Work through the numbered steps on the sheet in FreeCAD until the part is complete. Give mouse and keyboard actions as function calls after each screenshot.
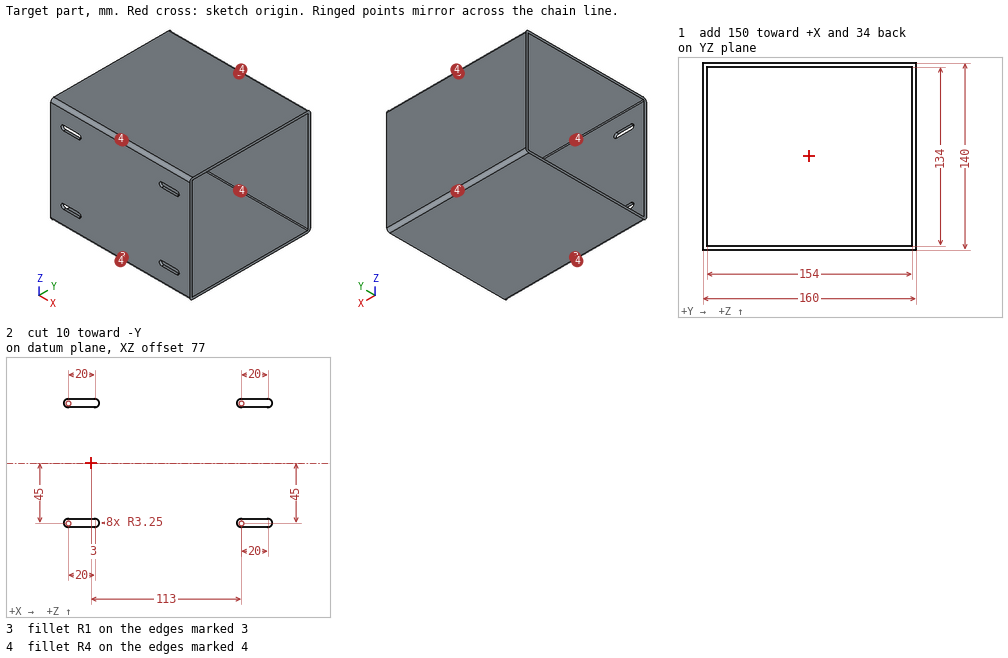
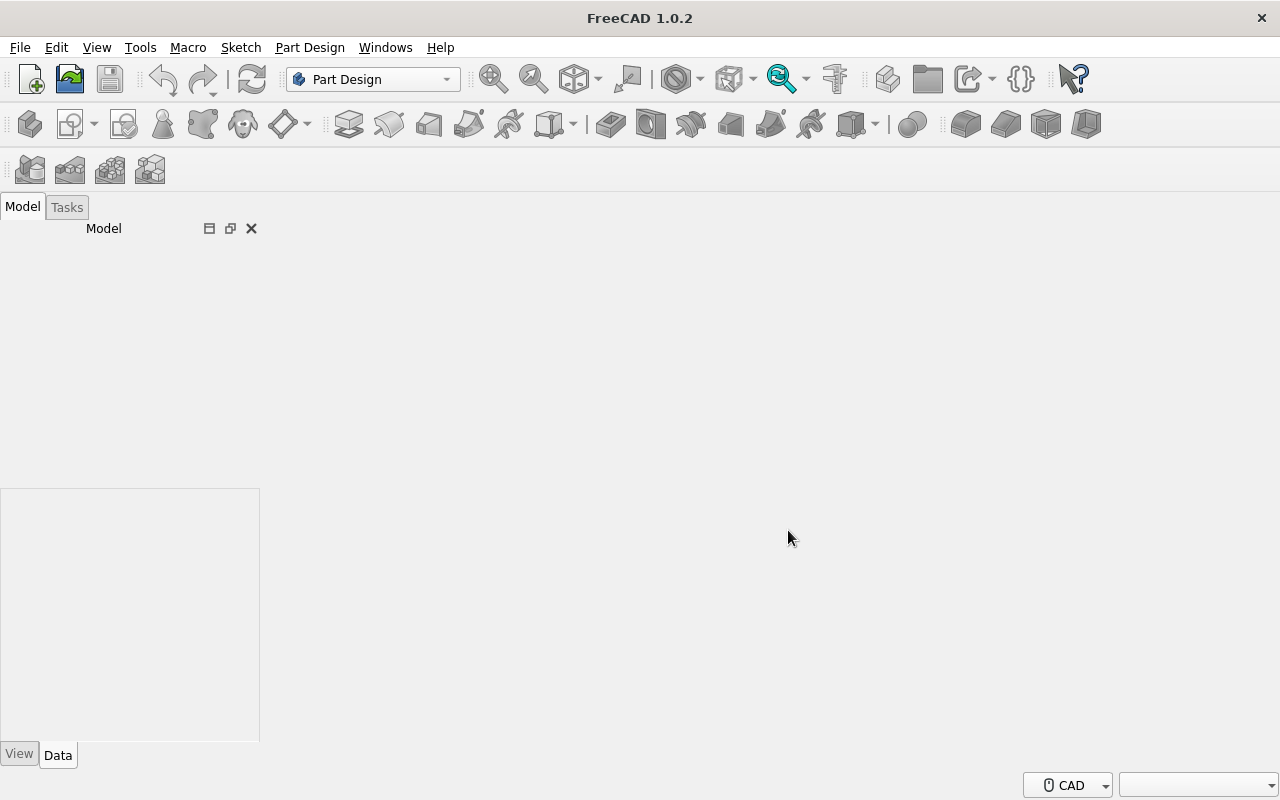
click(30, 80)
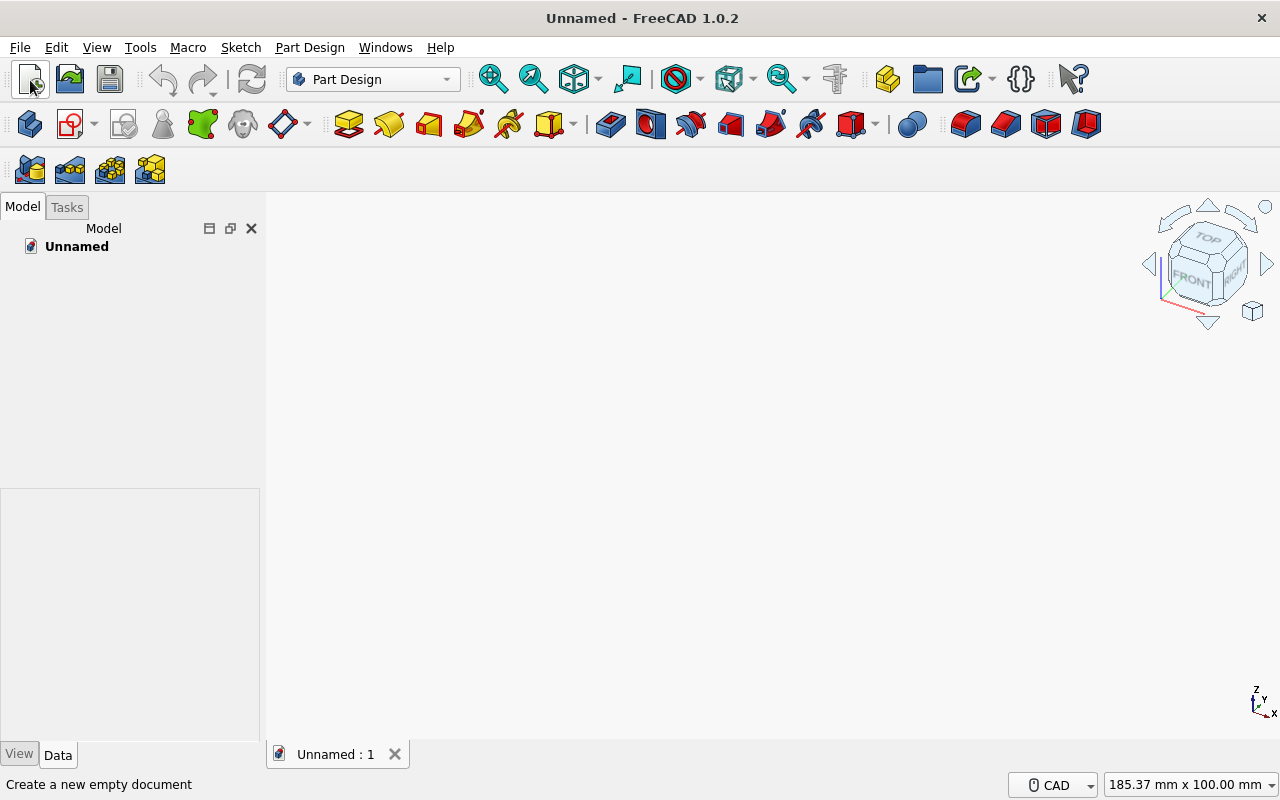
click(70, 124)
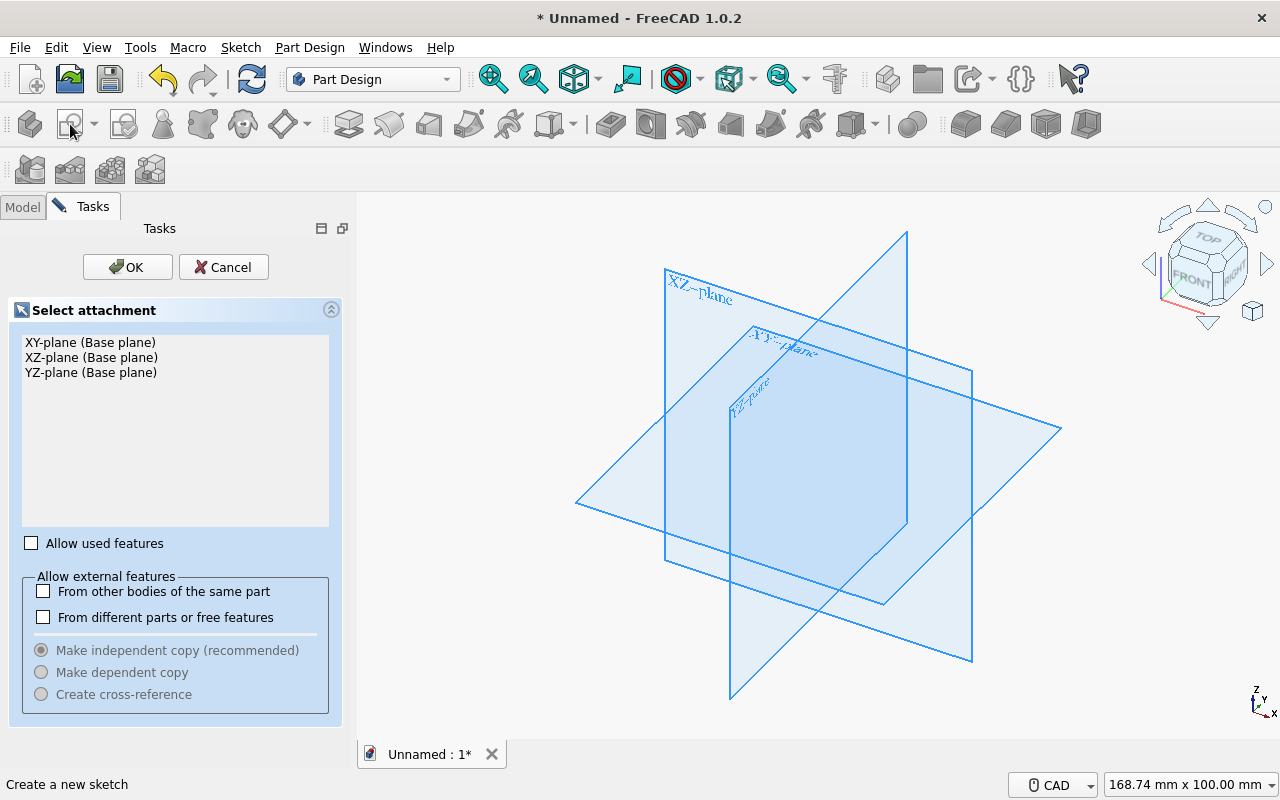
click(82, 372)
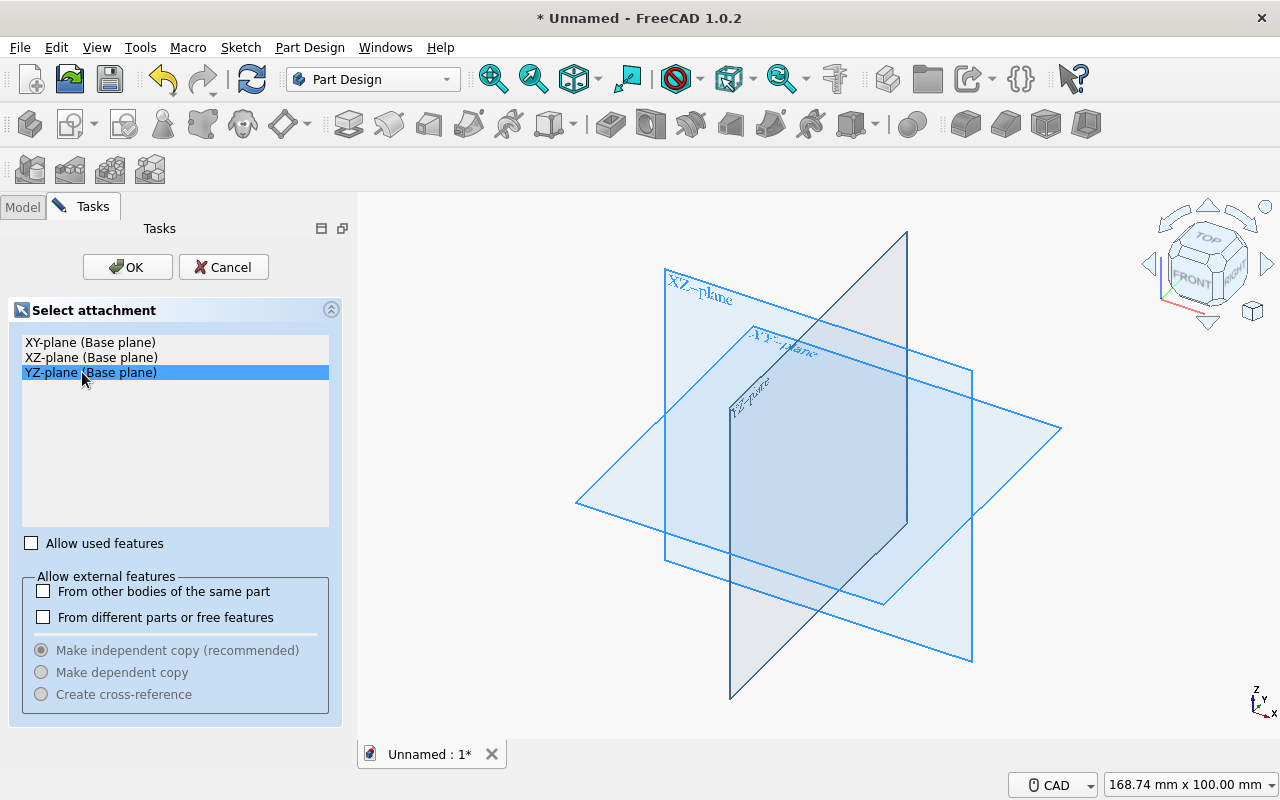
click(128, 267)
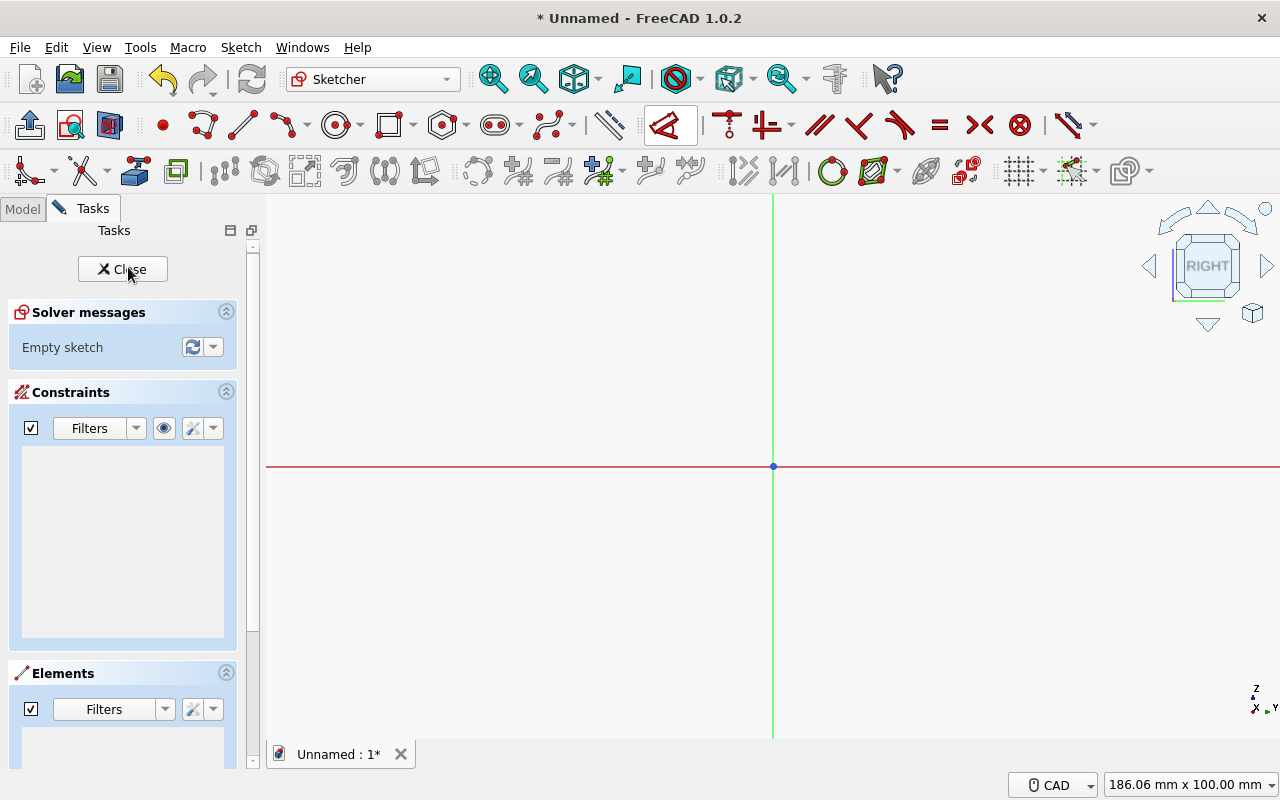
scroll(649, 466, down, 4)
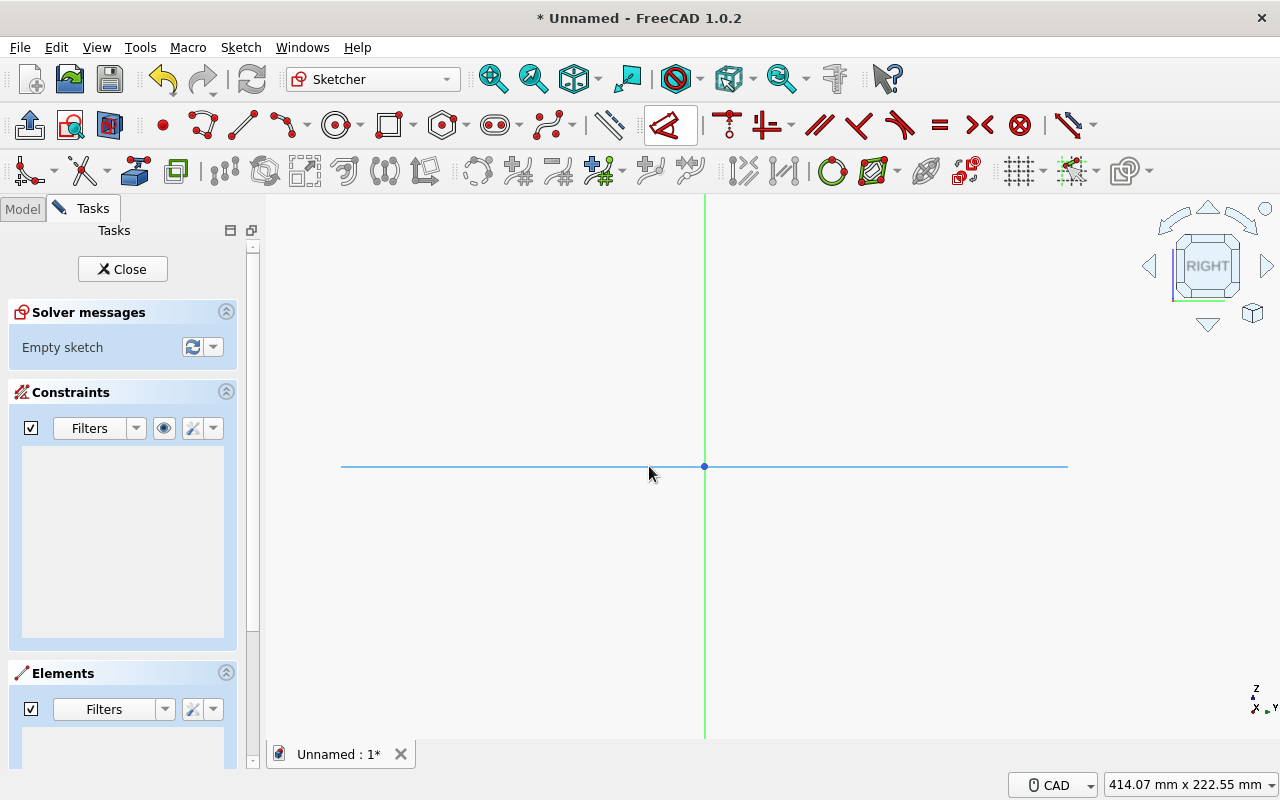
key(g)
key(v)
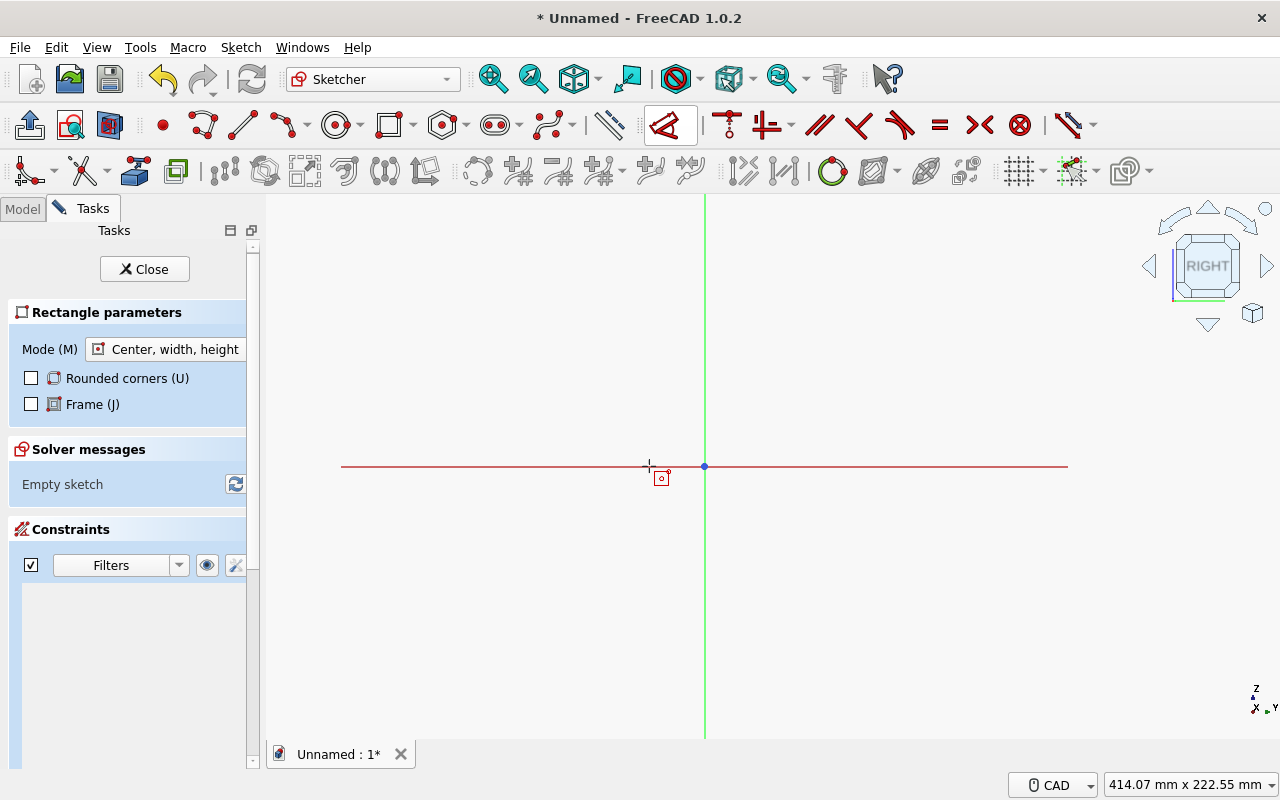
click(705, 466)
move(901, 295)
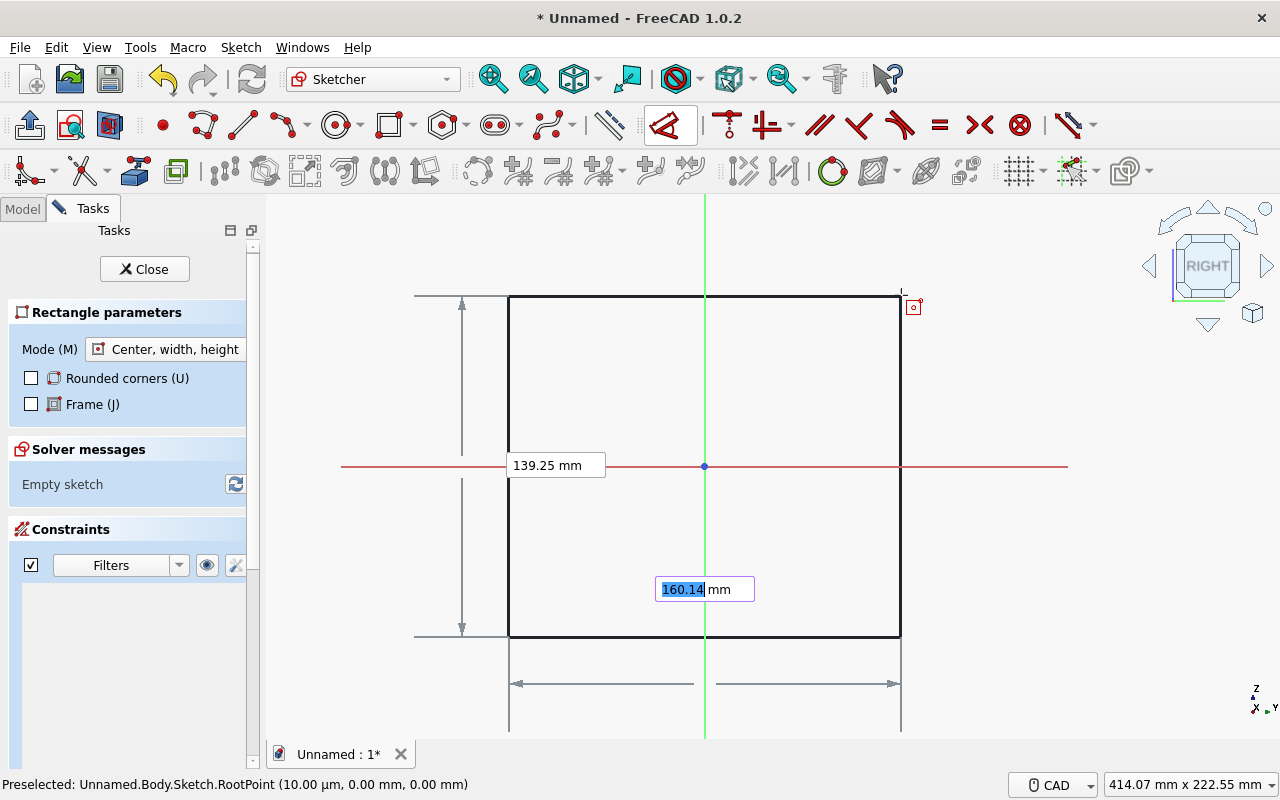
text(160)
key(Tab)
text(140)
key(Return)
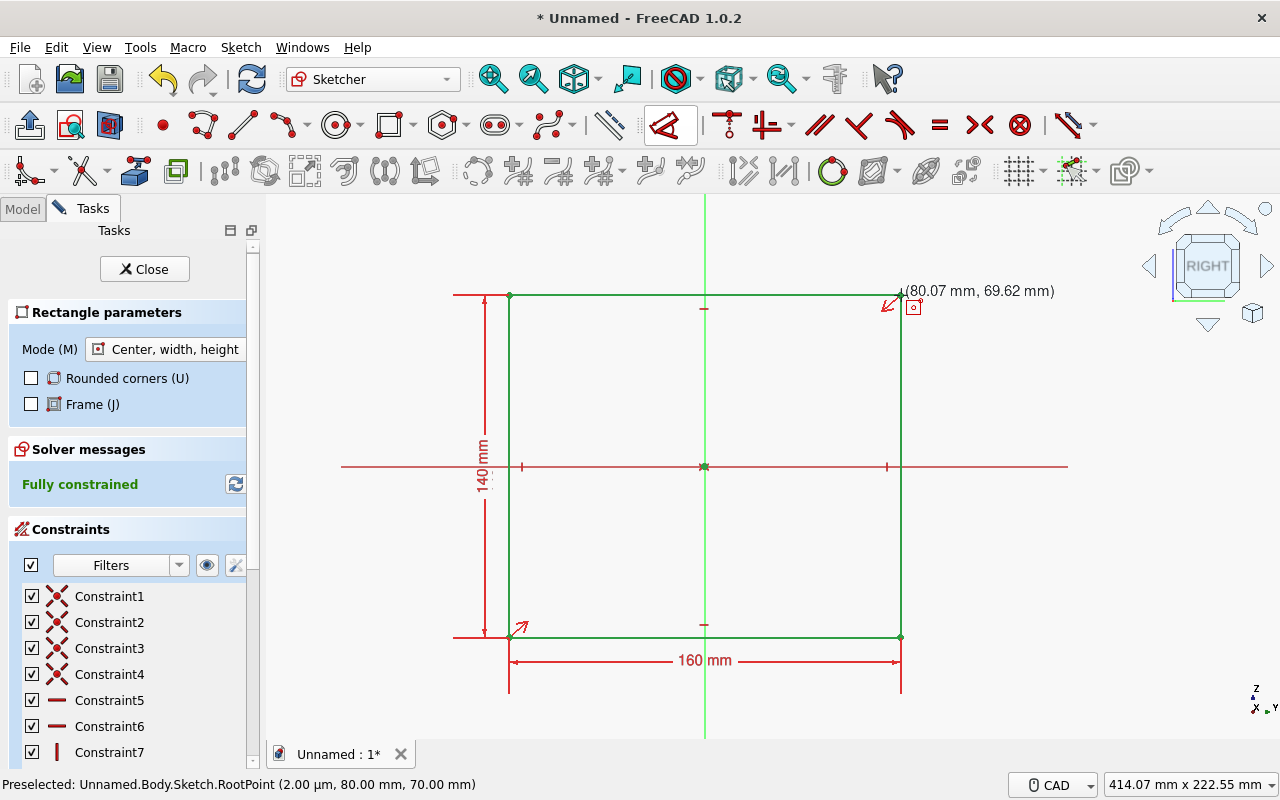
click(705, 466)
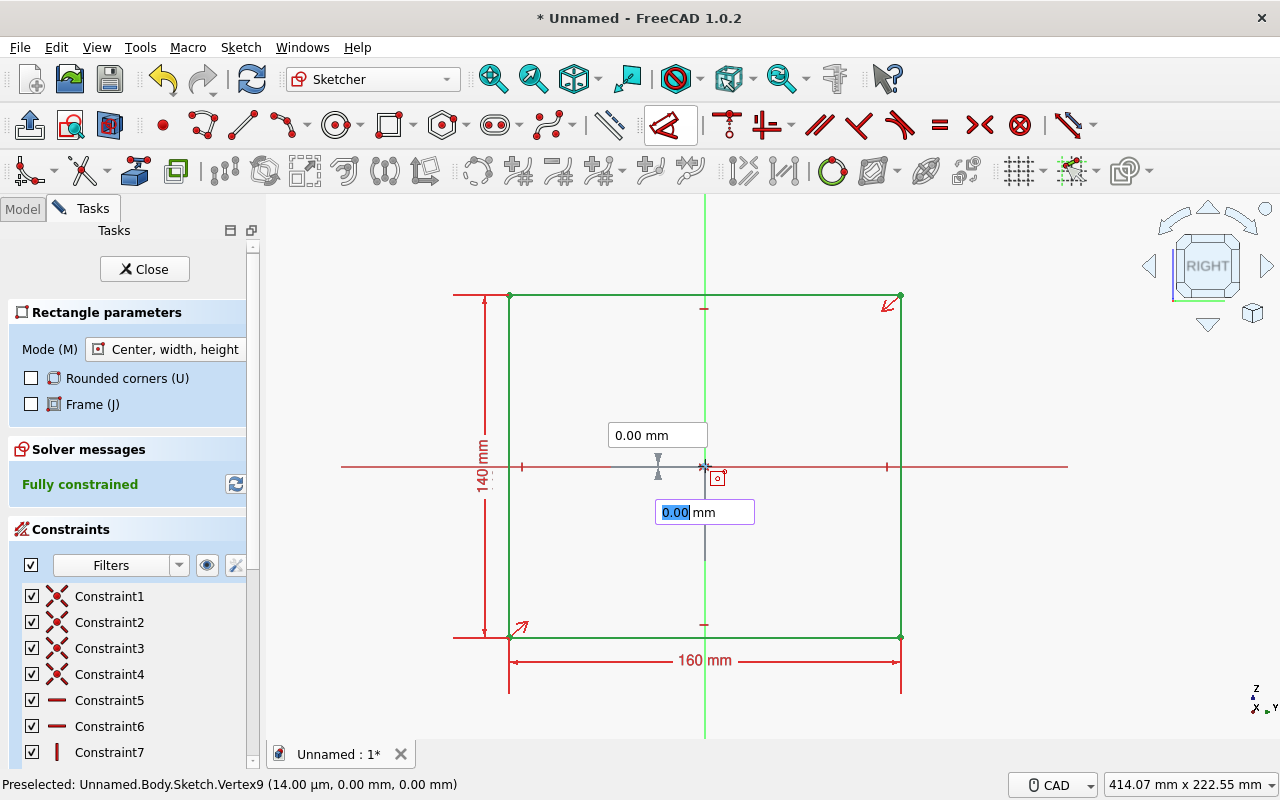
scroll(893, 302, up, 4)
move(893, 303)